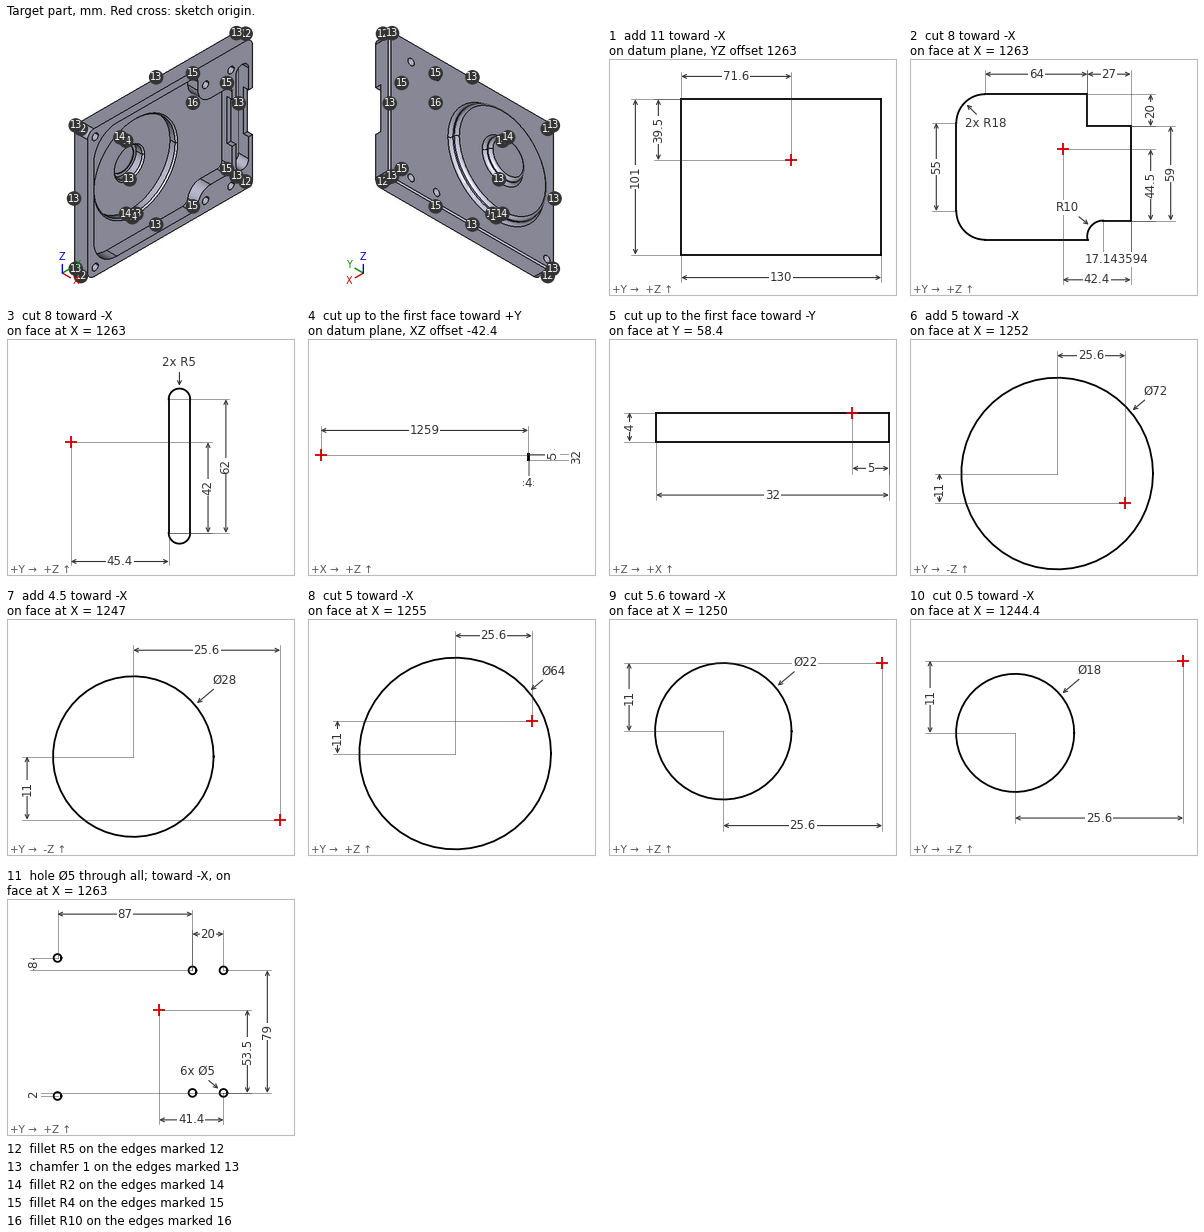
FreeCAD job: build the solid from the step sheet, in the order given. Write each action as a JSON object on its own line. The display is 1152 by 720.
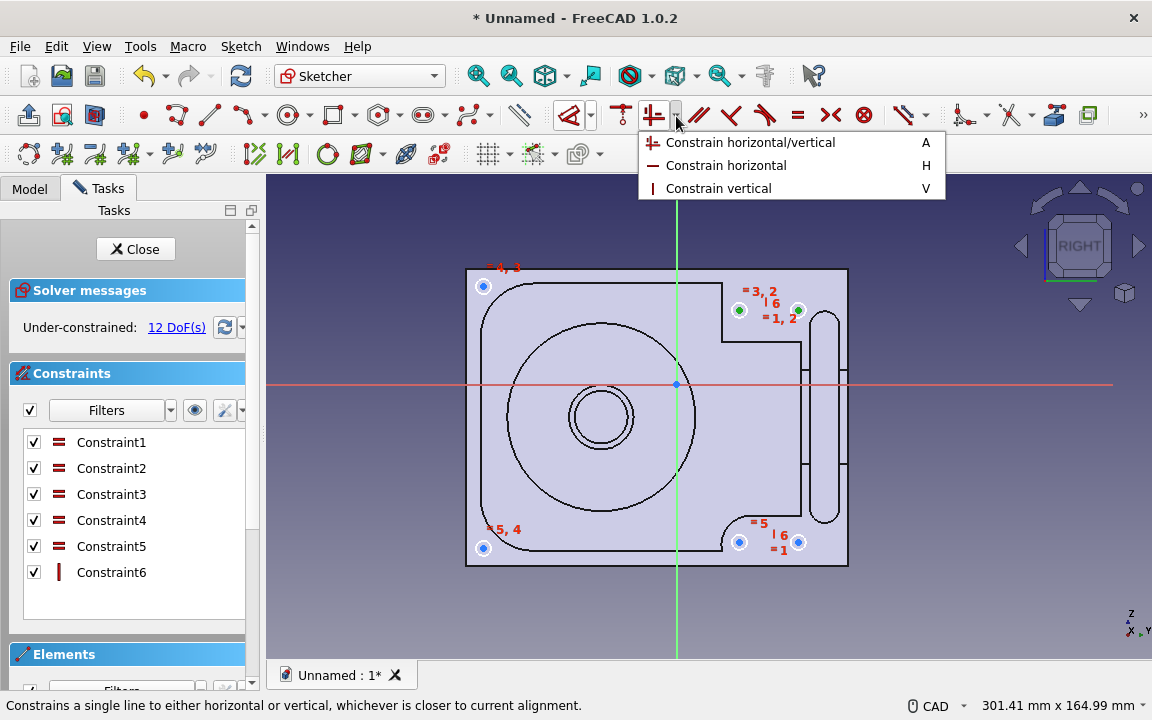
{"action": "left_click", "coordinate": [792, 166]}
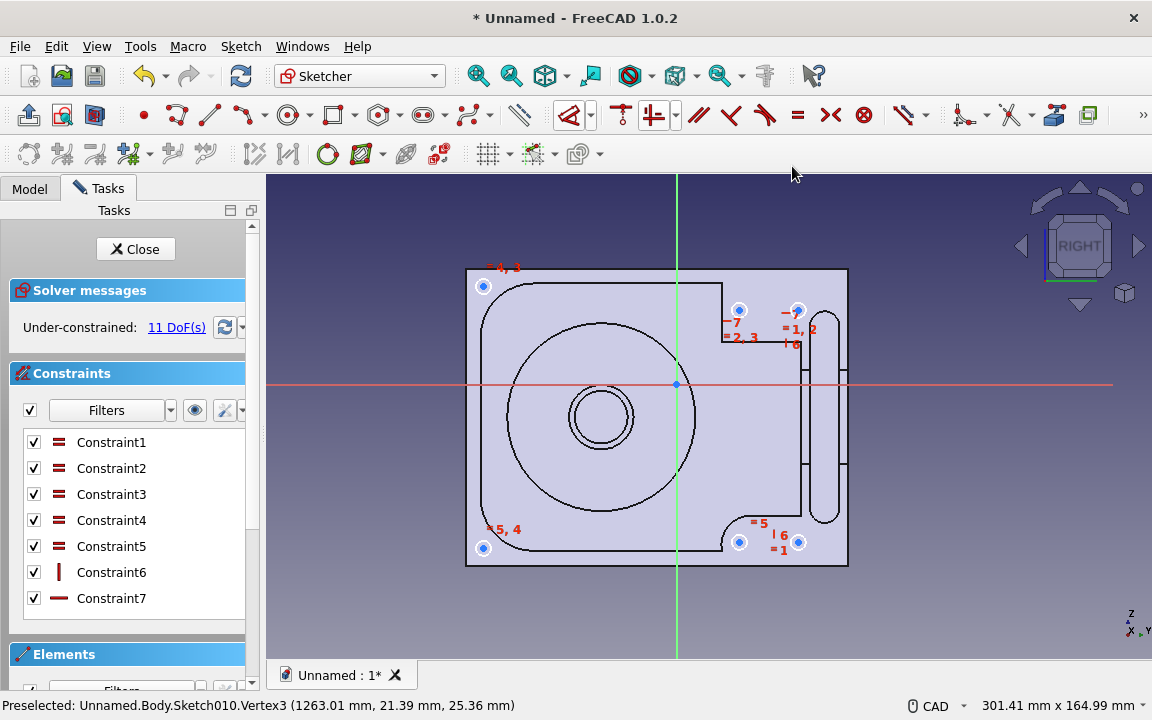
{"action": "left_click", "coordinate": [484, 287]}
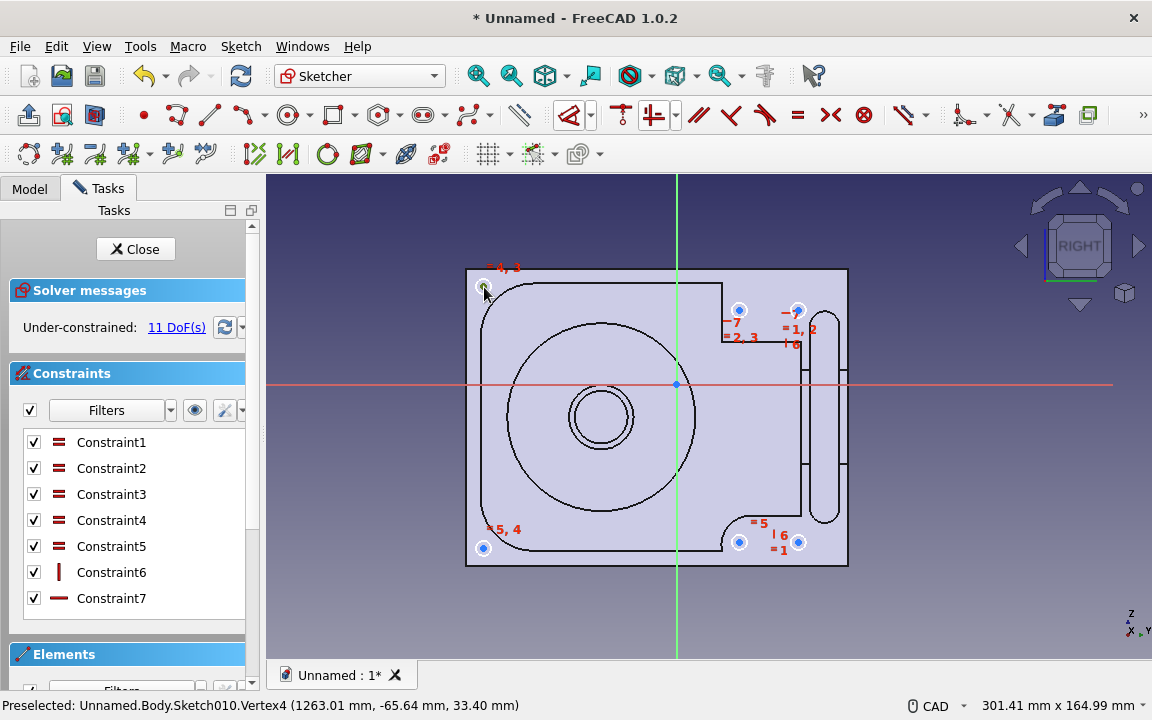
{"action": "left_click", "coordinate": [484, 548]}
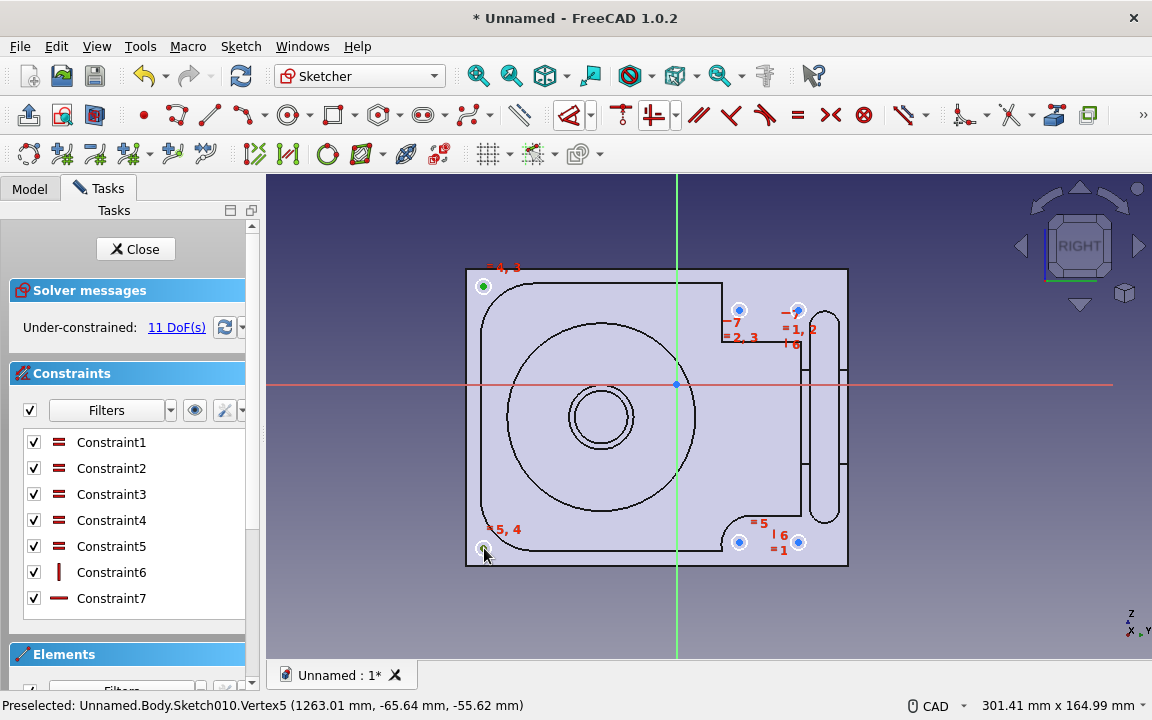
{"action": "key", "text": "v"}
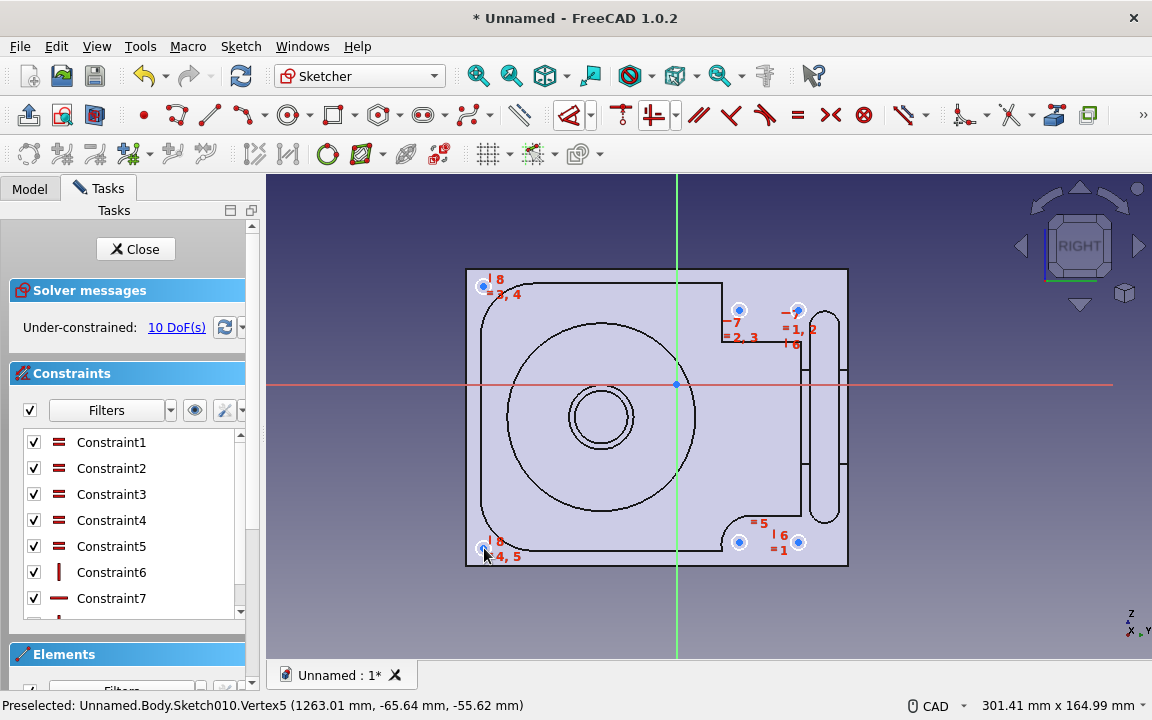
{"action": "left_click", "coordinate": [739, 310]}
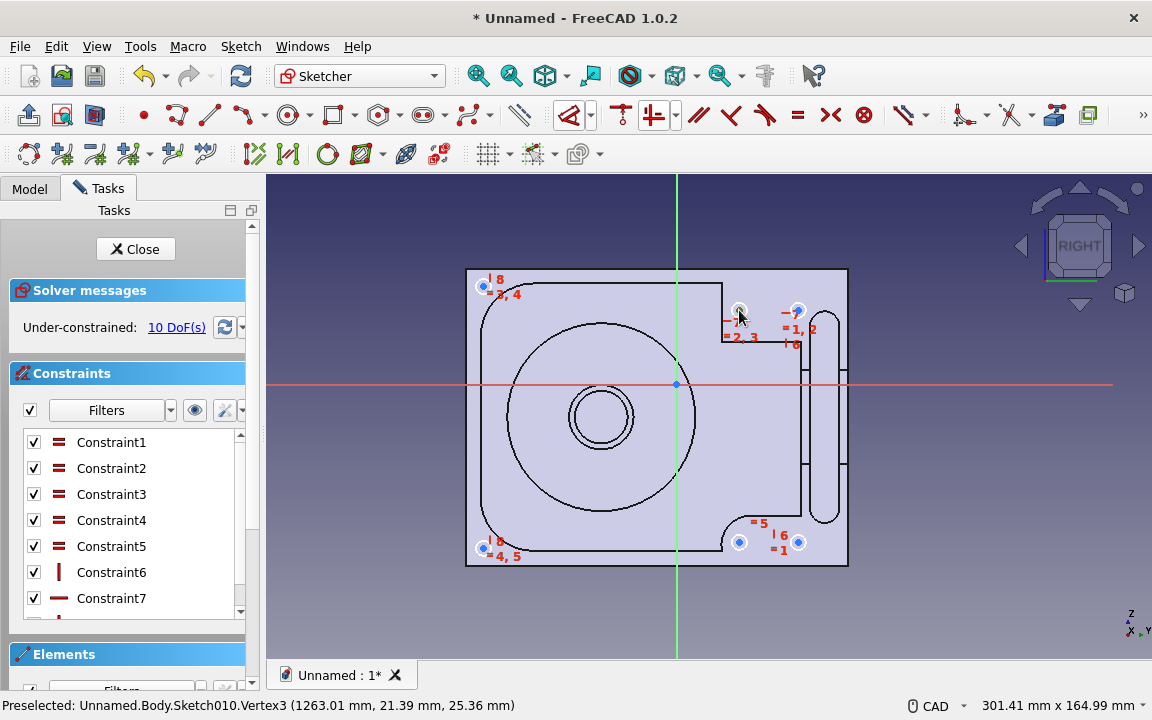
{"action": "left_click", "coordinate": [739, 542]}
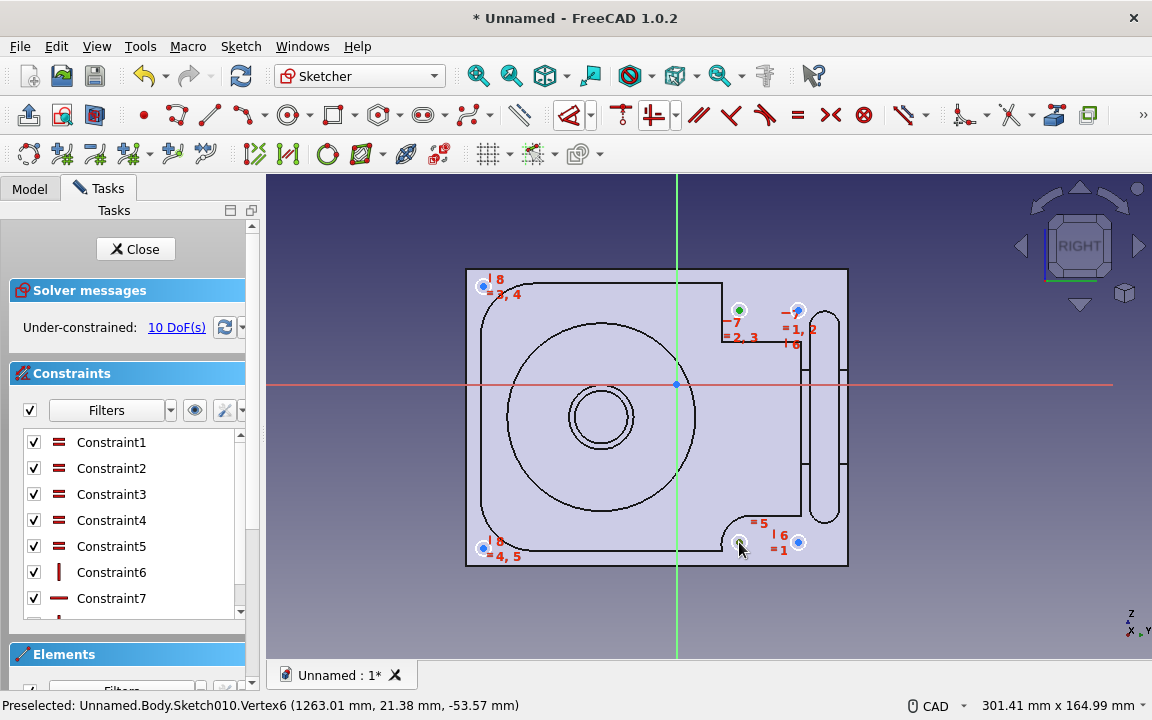
{"action": "key", "text": "v"}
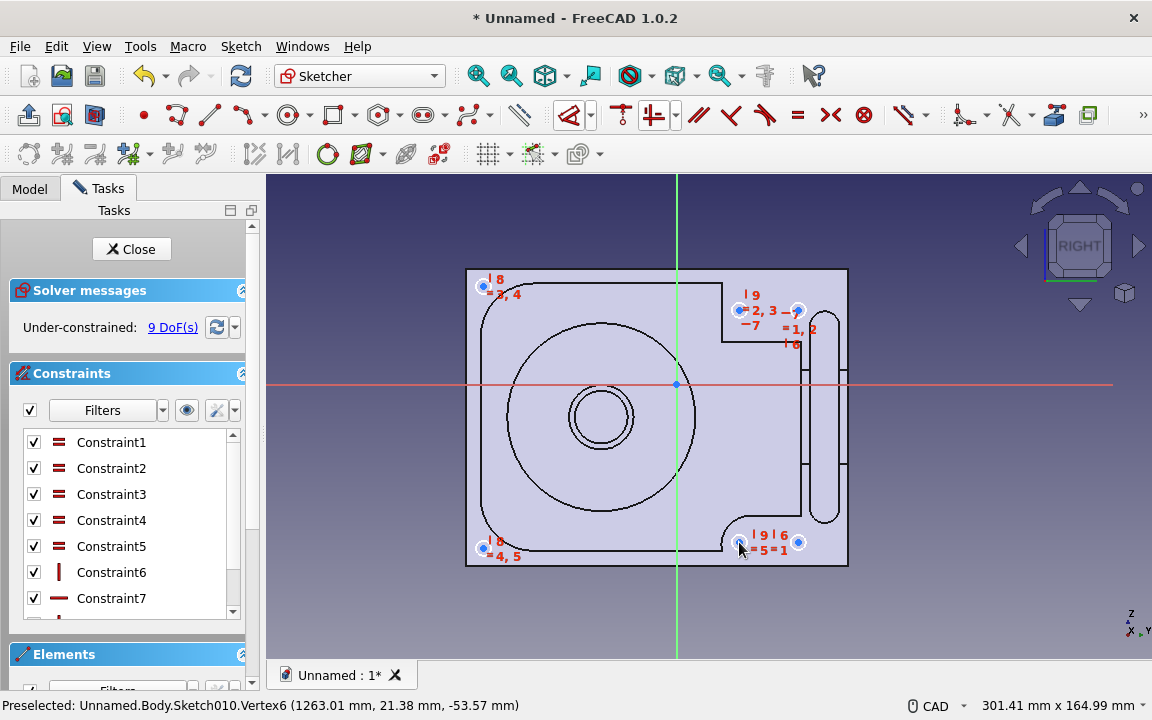
{"action": "left_click", "coordinate": [798, 543]}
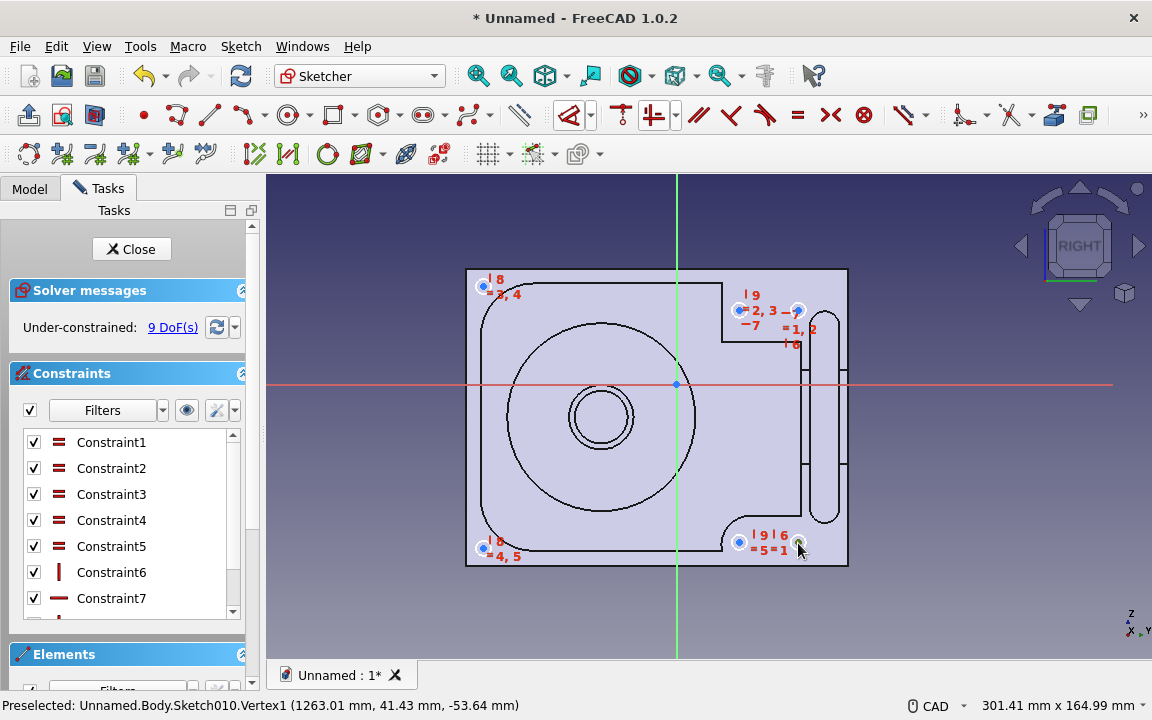
{"action": "left_click", "coordinate": [739, 542]}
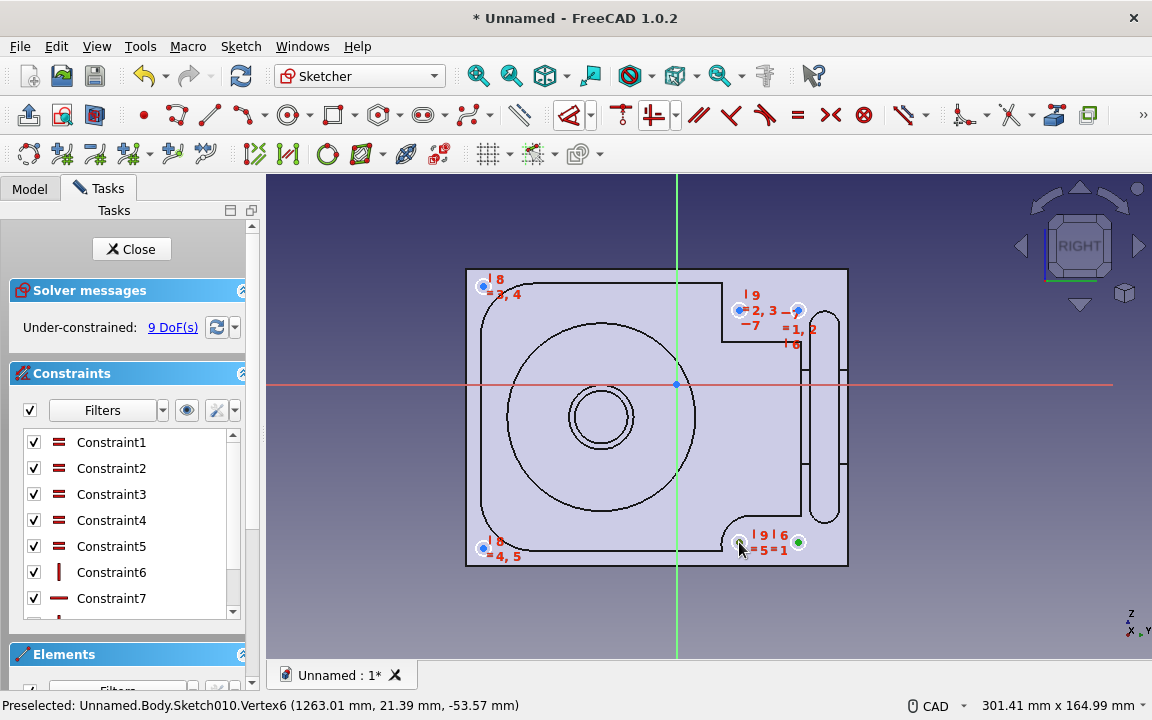
{"action": "left_click", "coordinate": [676, 116]}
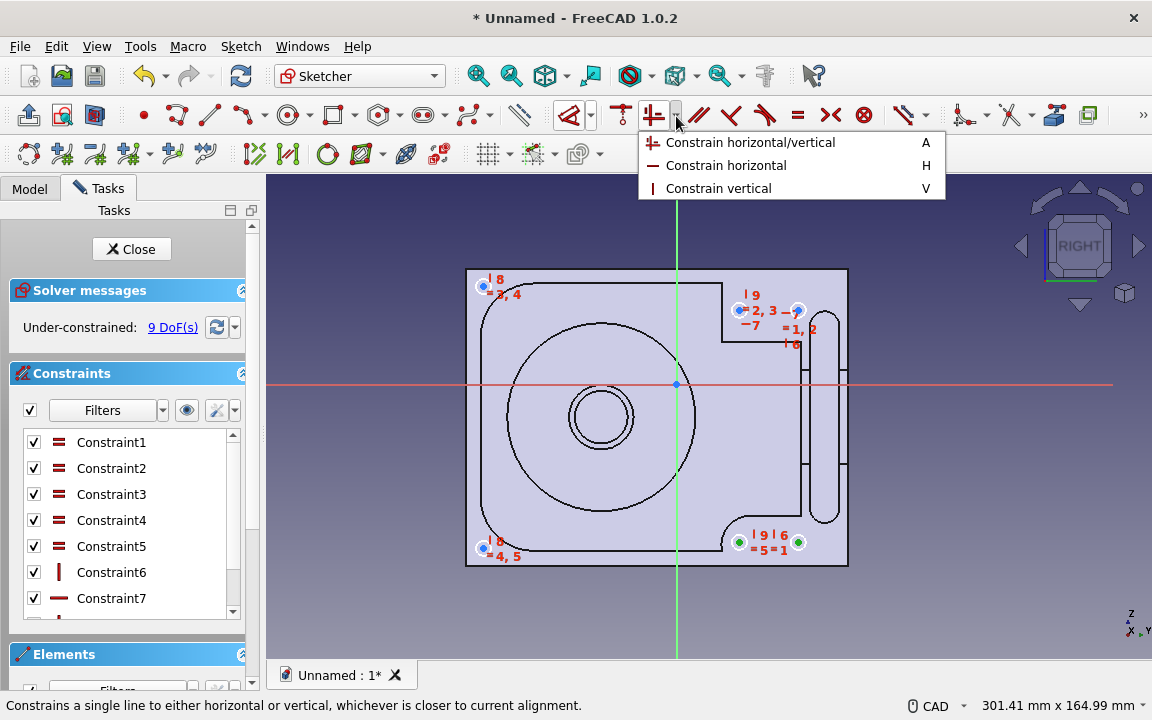
{"action": "left_click", "coordinate": [792, 166]}